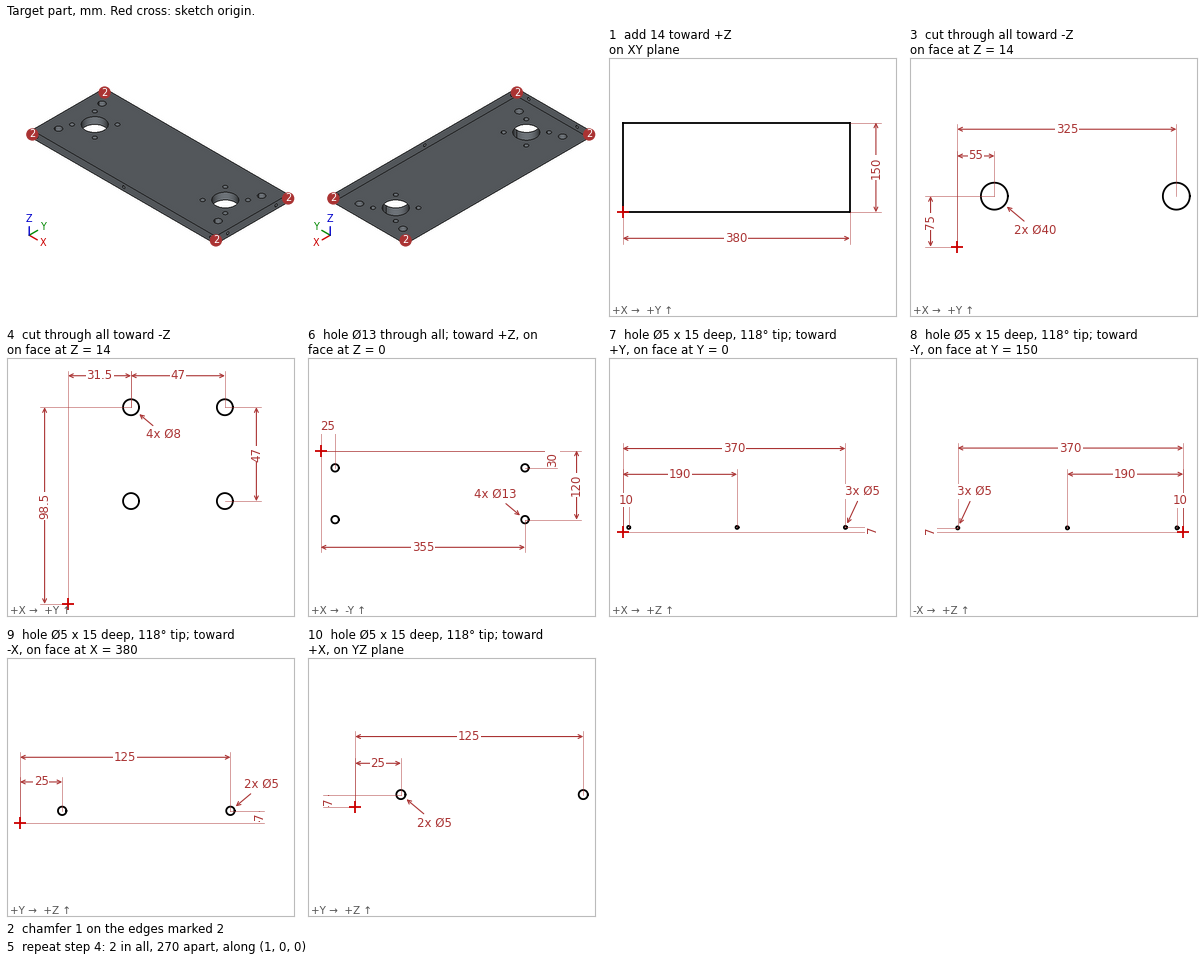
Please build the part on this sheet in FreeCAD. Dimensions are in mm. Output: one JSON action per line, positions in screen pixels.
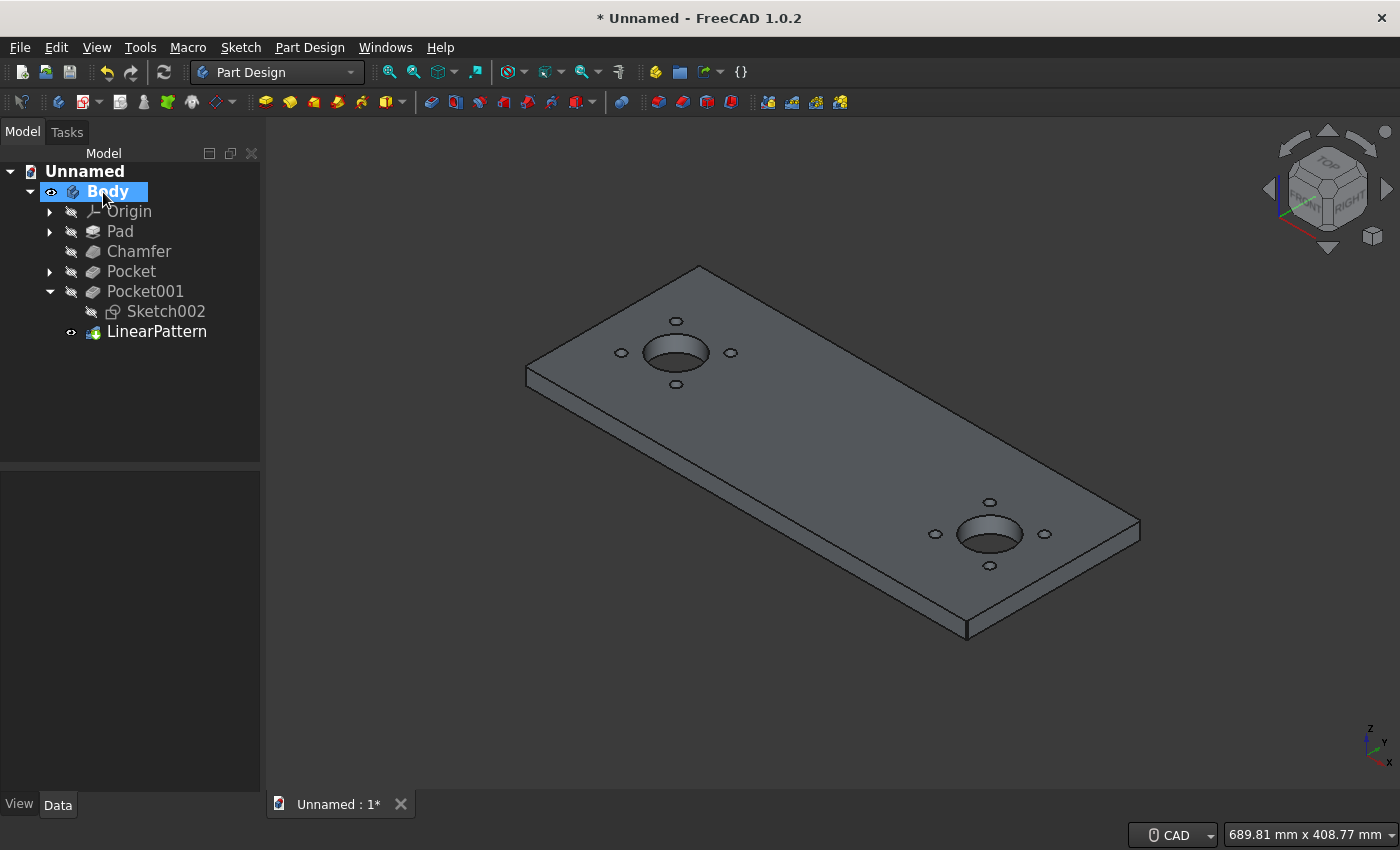
{"action": "key", "text": "5"}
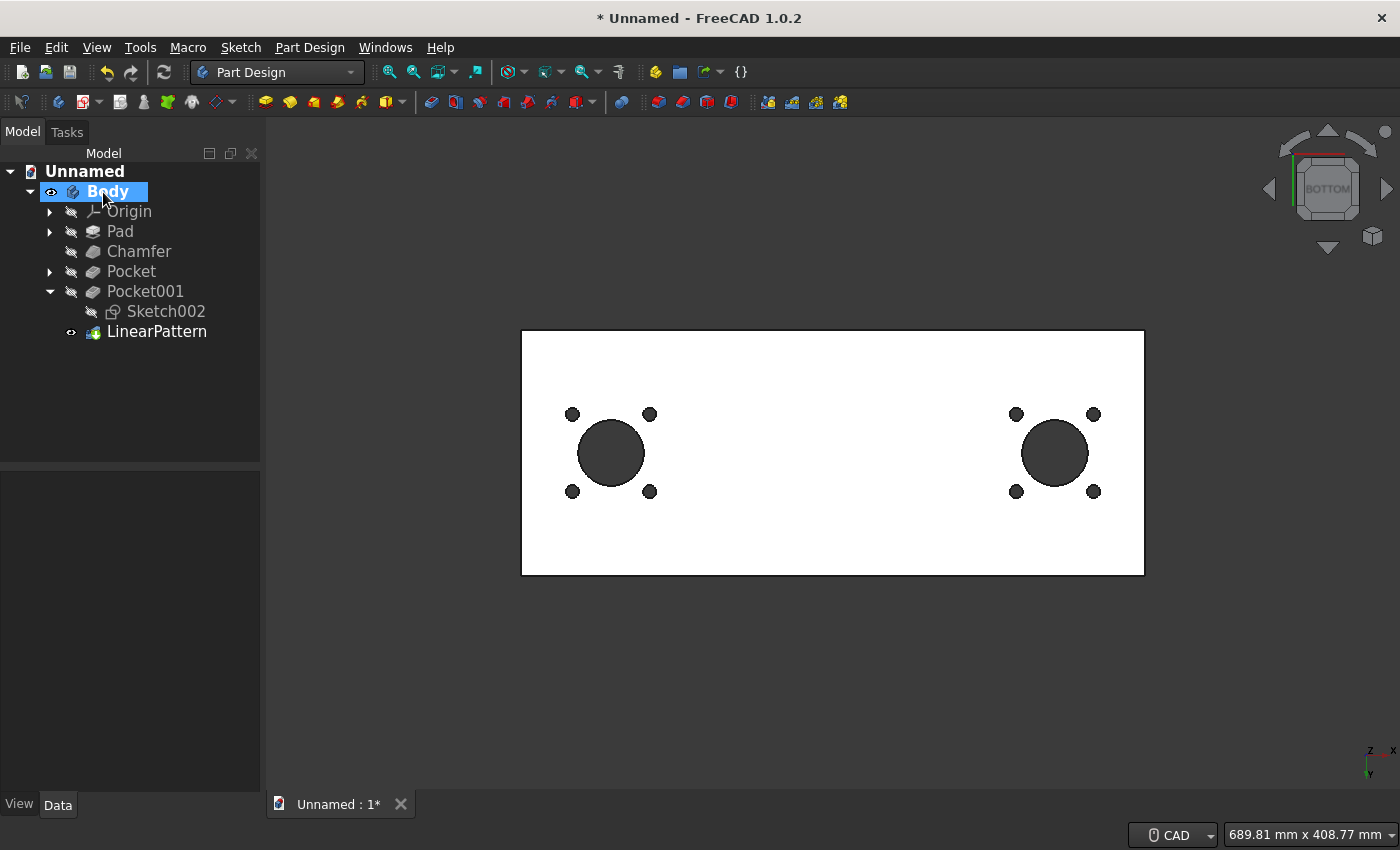
{"action": "left_click", "coordinate": [833, 452]}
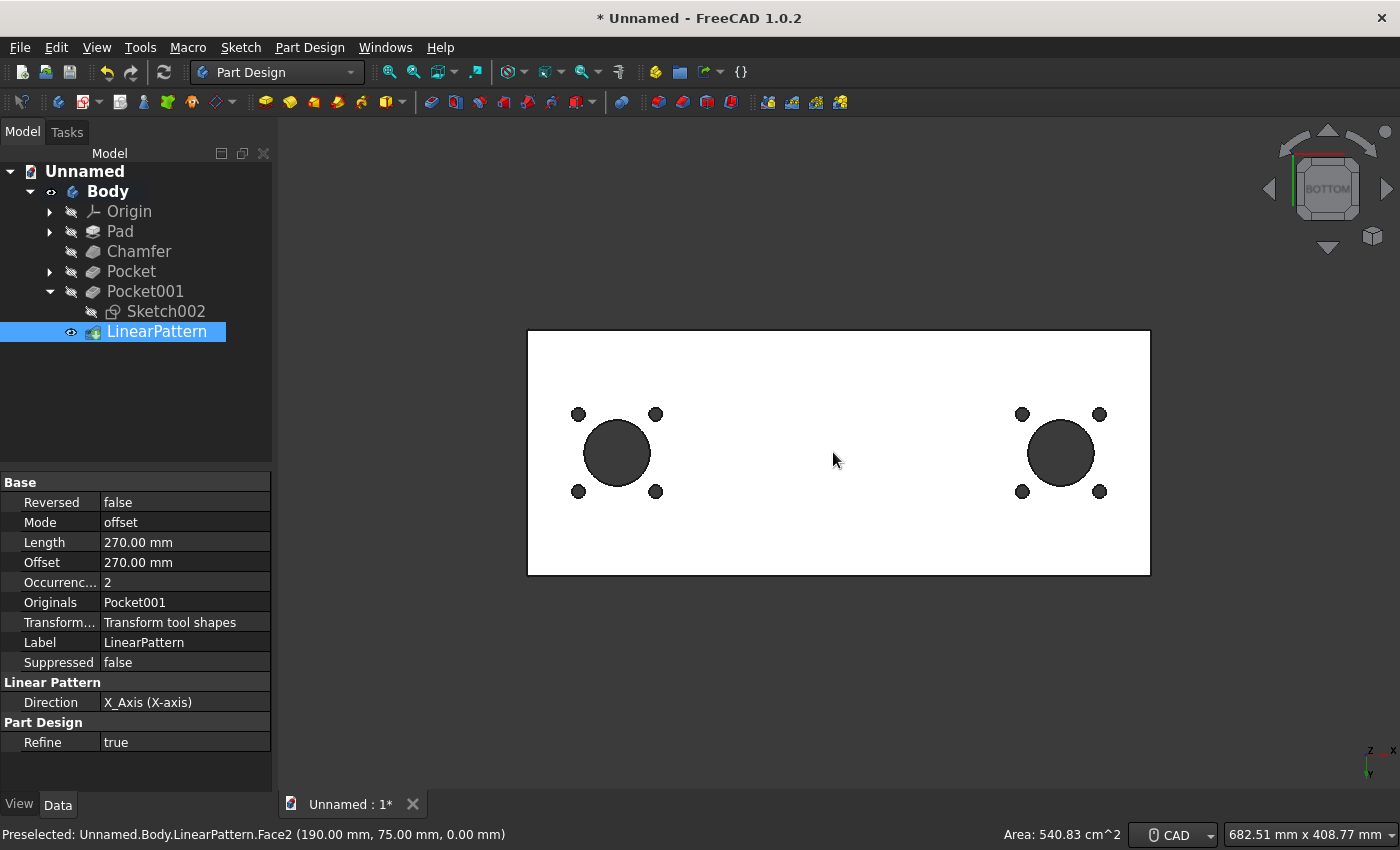
{"action": "left_click", "coordinate": [84, 102]}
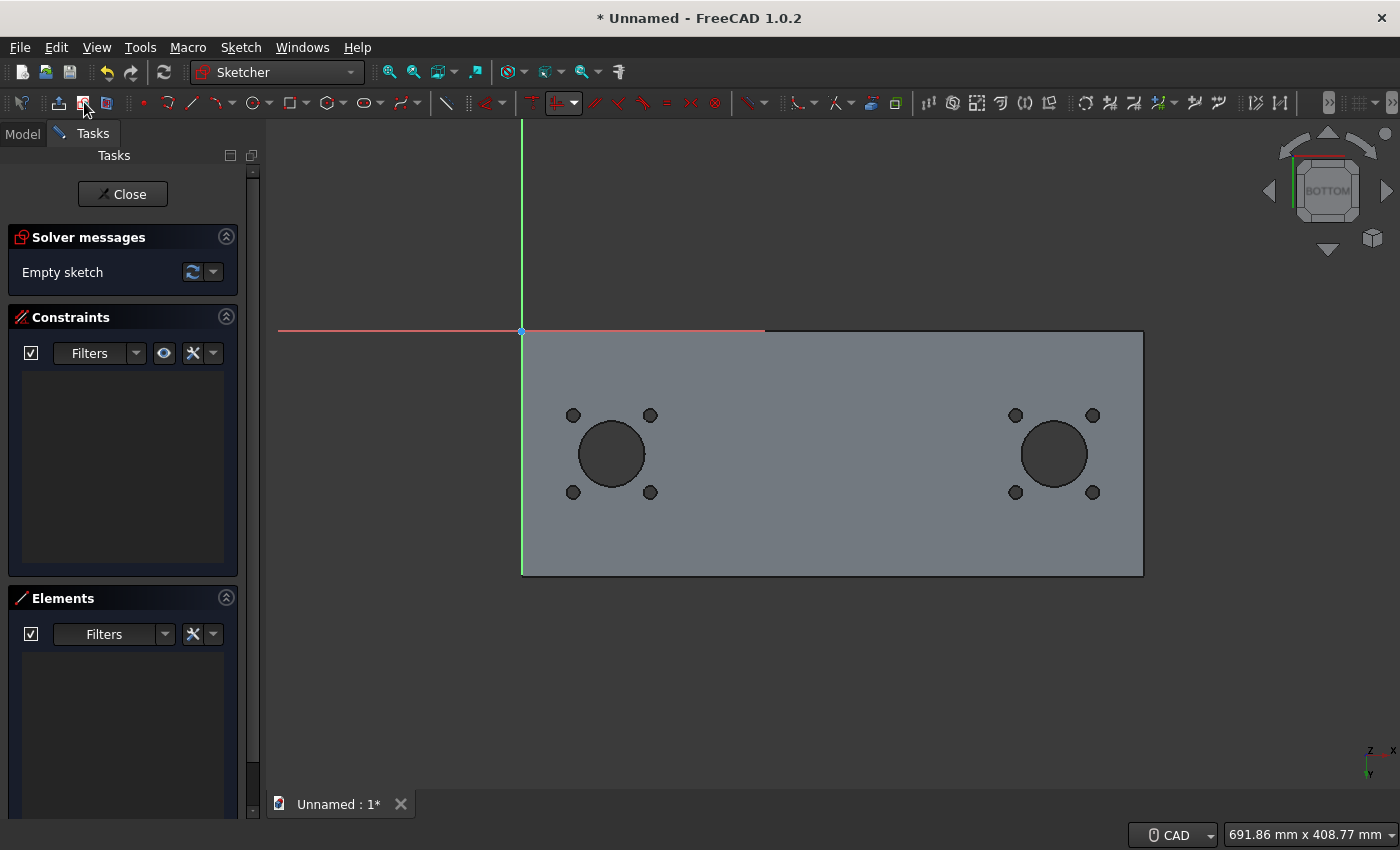
{"action": "key", "text": "g c"}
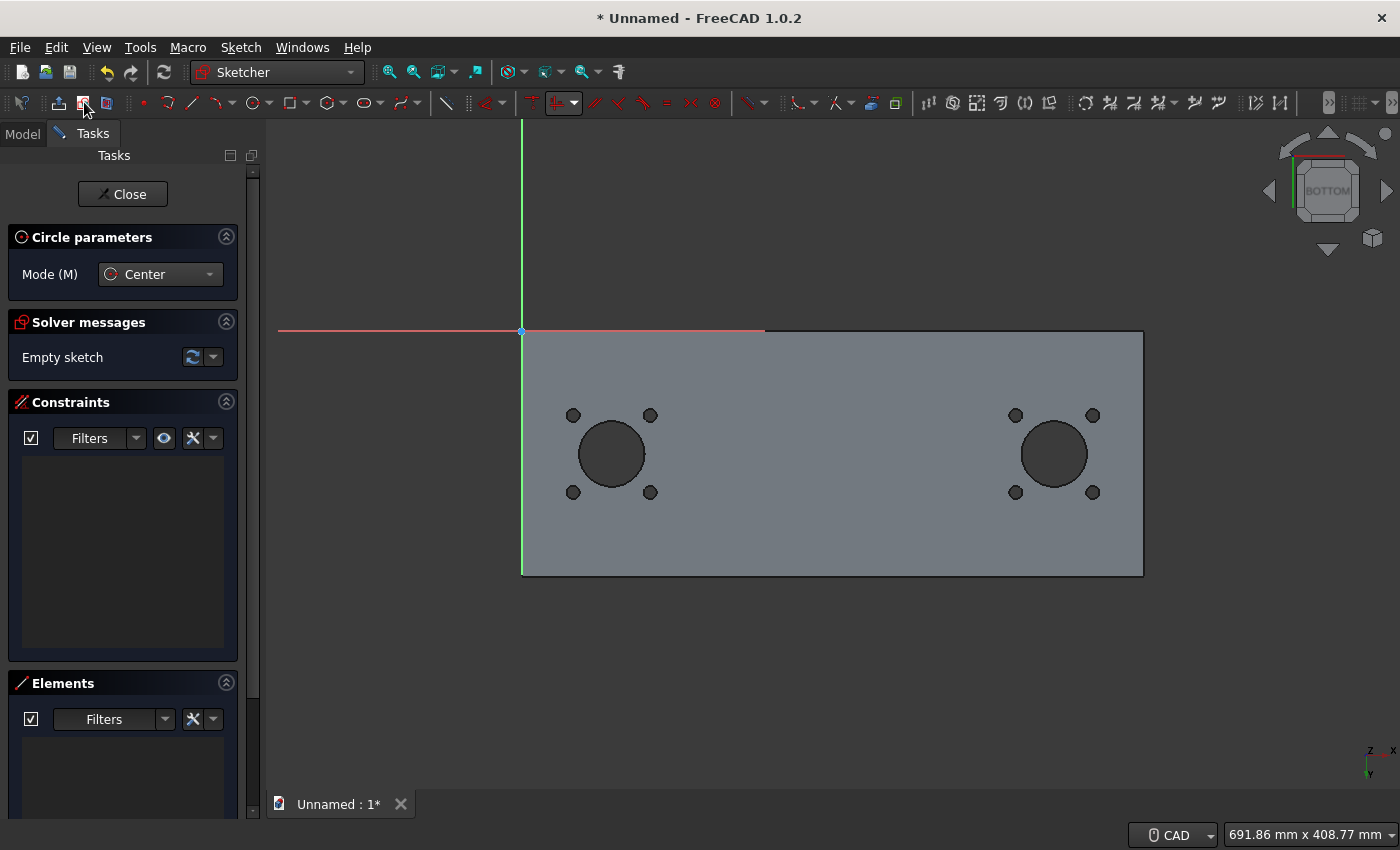
{"action": "scroll", "coordinate": [1103, 528], "scroll_direction": "up", "scroll_amount": 4}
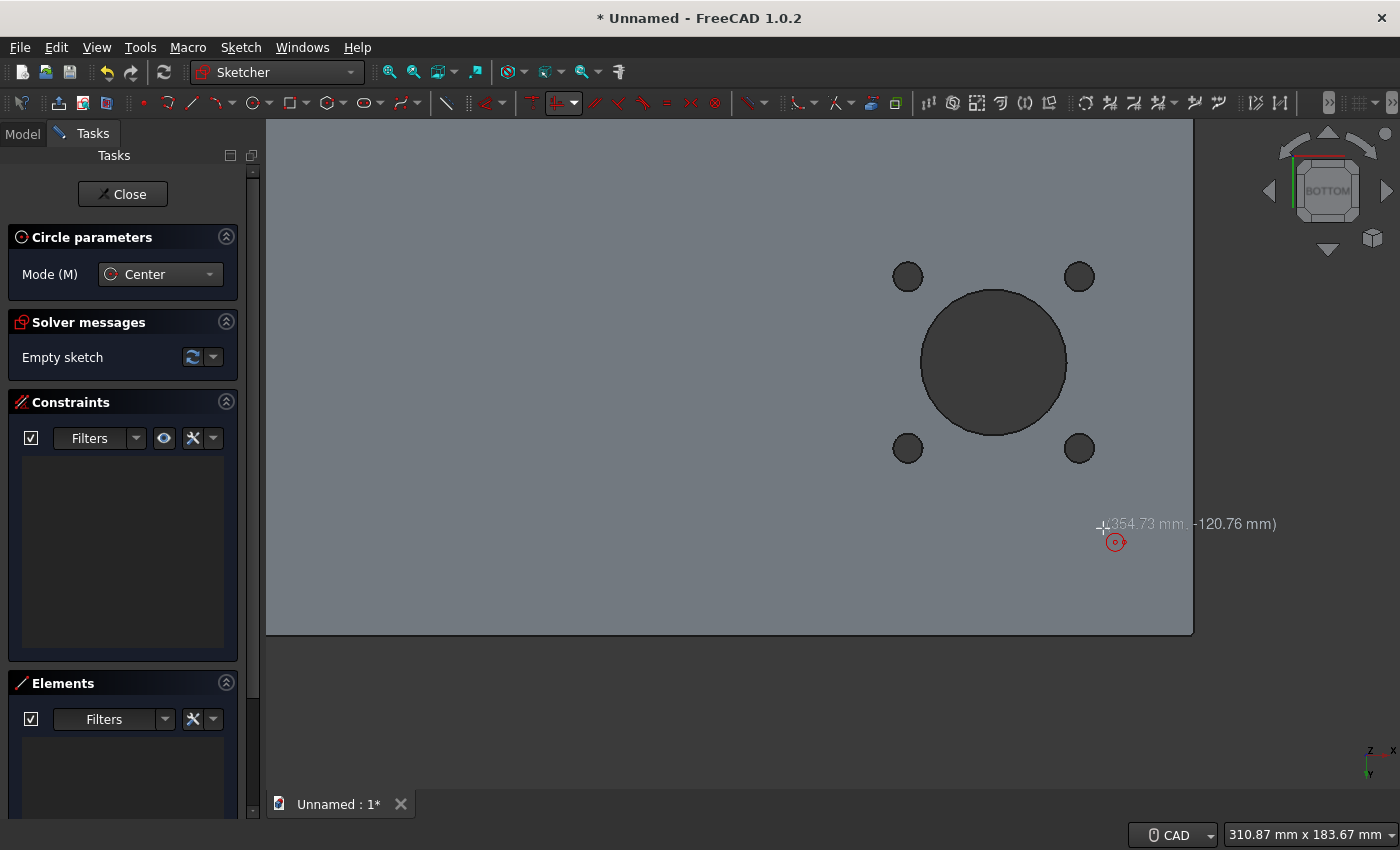
{"action": "left_click", "coordinate": [1103, 527]}
{"action": "mouse_move", "coordinate": [1120, 510]}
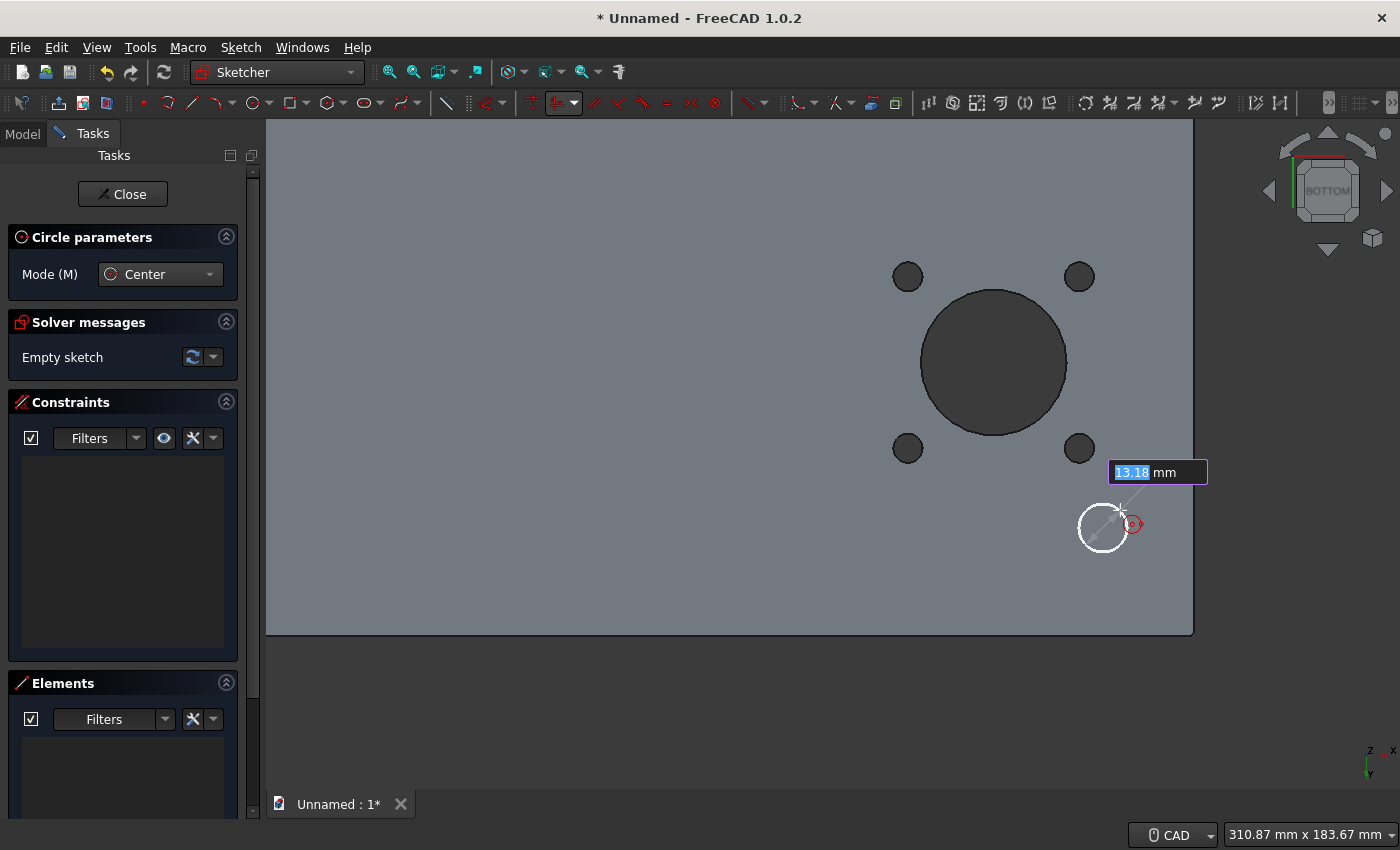
{"action": "type", "text": "13"}
{"action": "key", "text": "Return"}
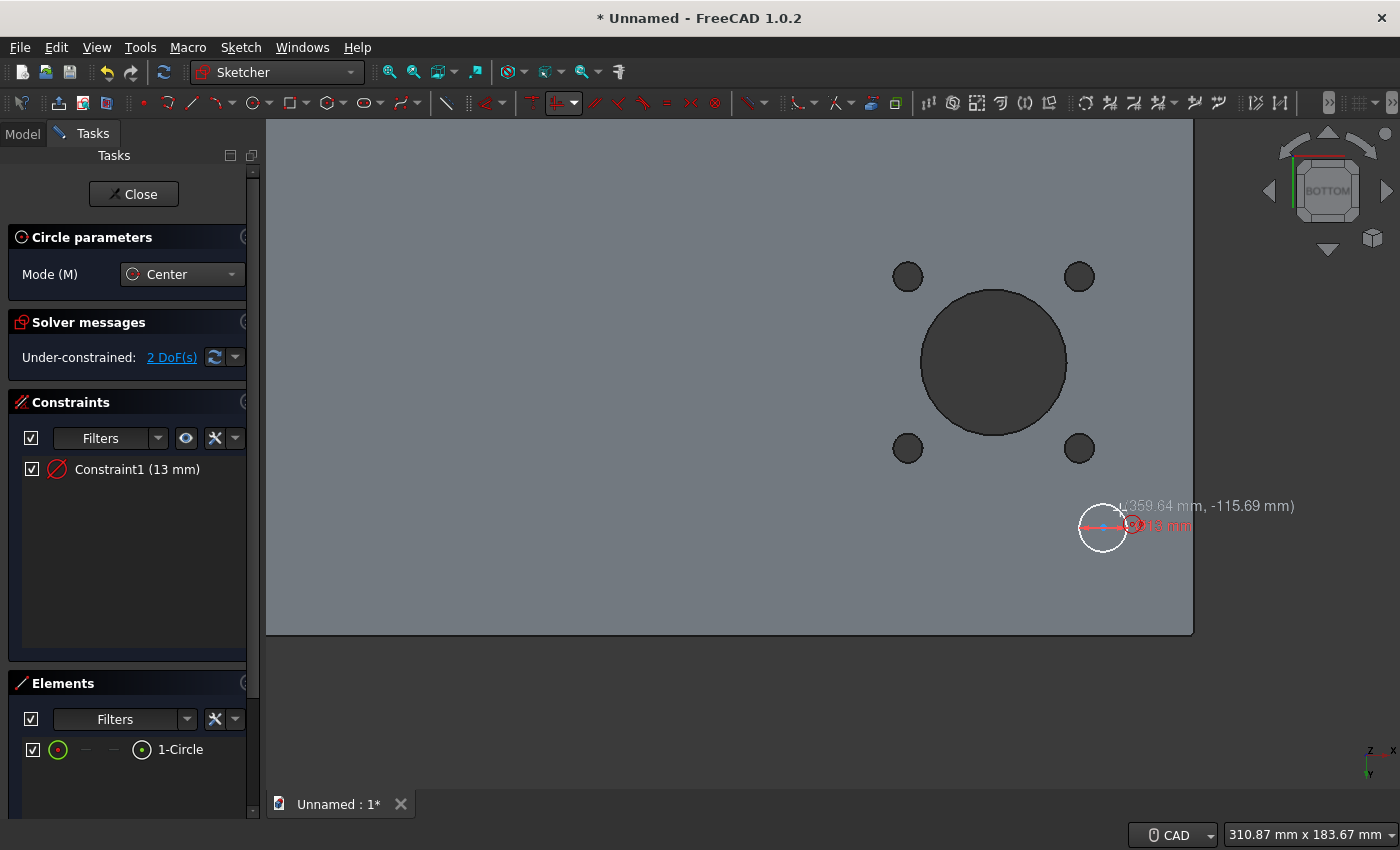
{"action": "left_click", "coordinate": [1103, 198]}
{"action": "mouse_move", "coordinate": [1120, 182]}